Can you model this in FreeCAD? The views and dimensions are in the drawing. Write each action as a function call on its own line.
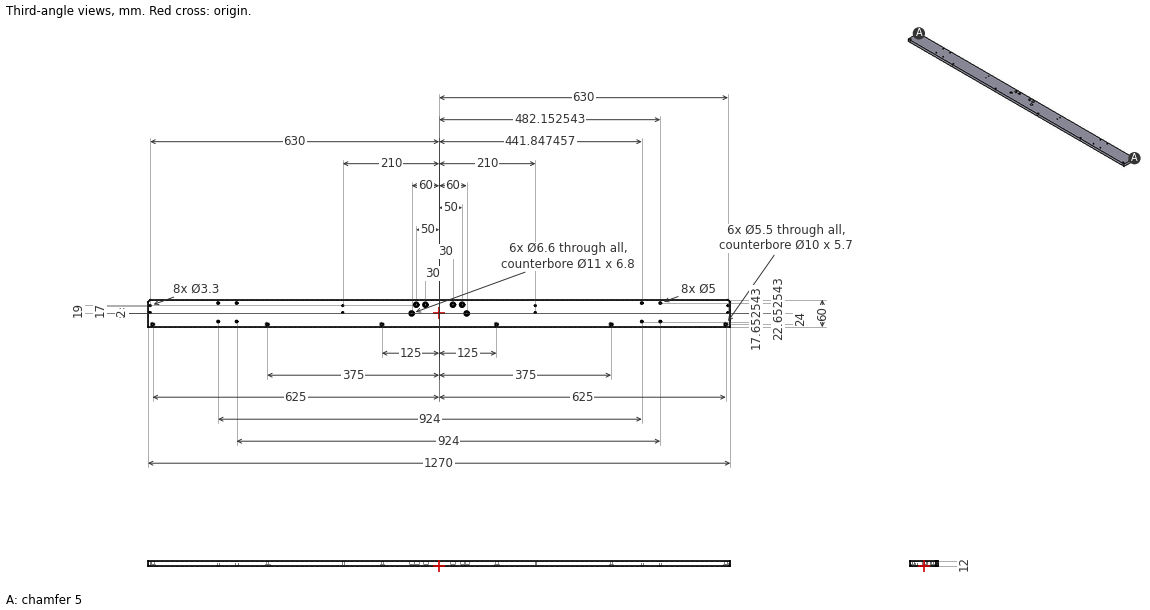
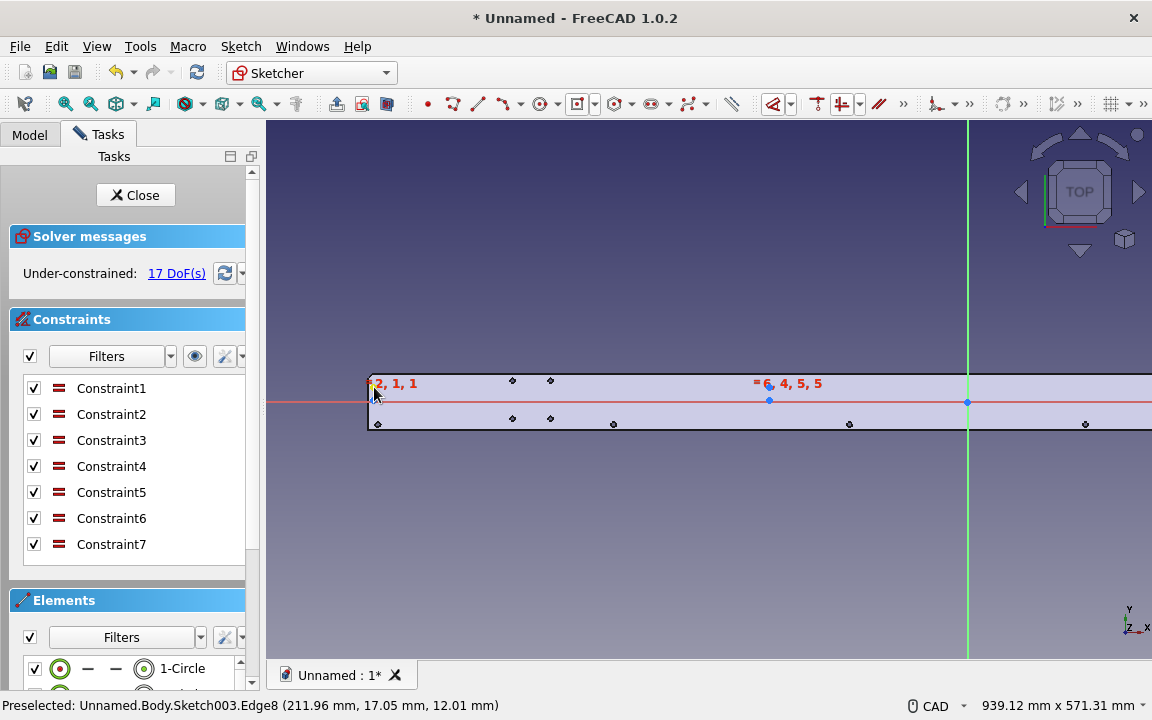
click(373, 387)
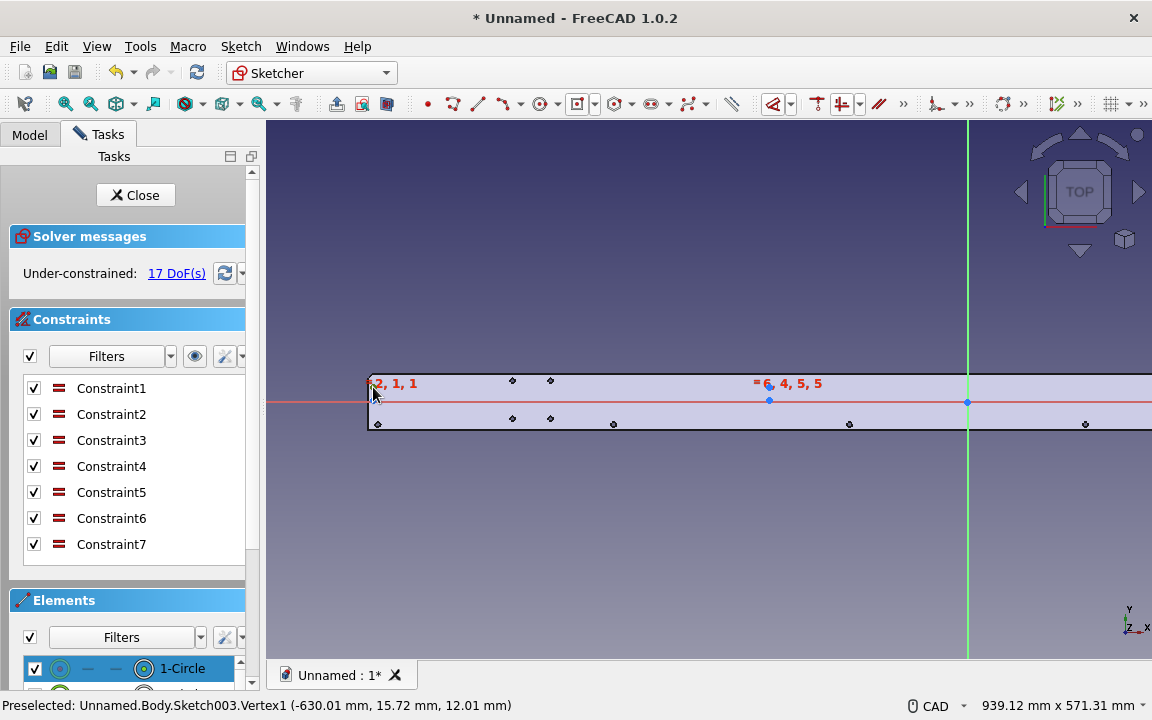
click(373, 400)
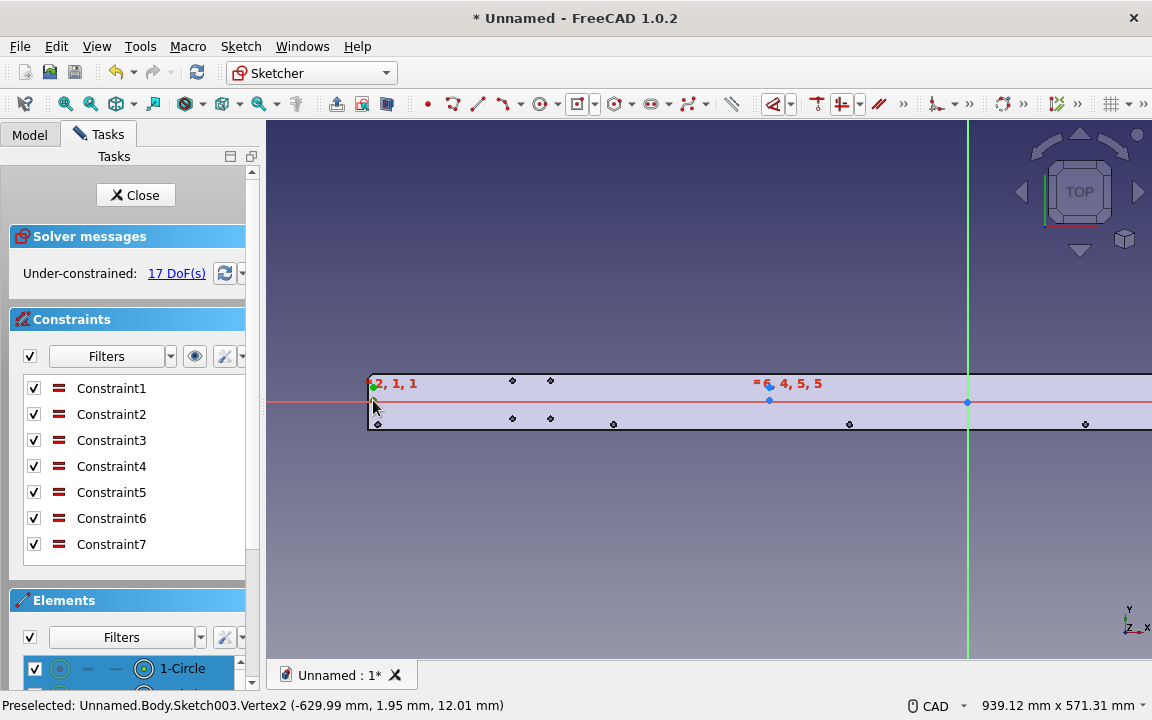
key(v)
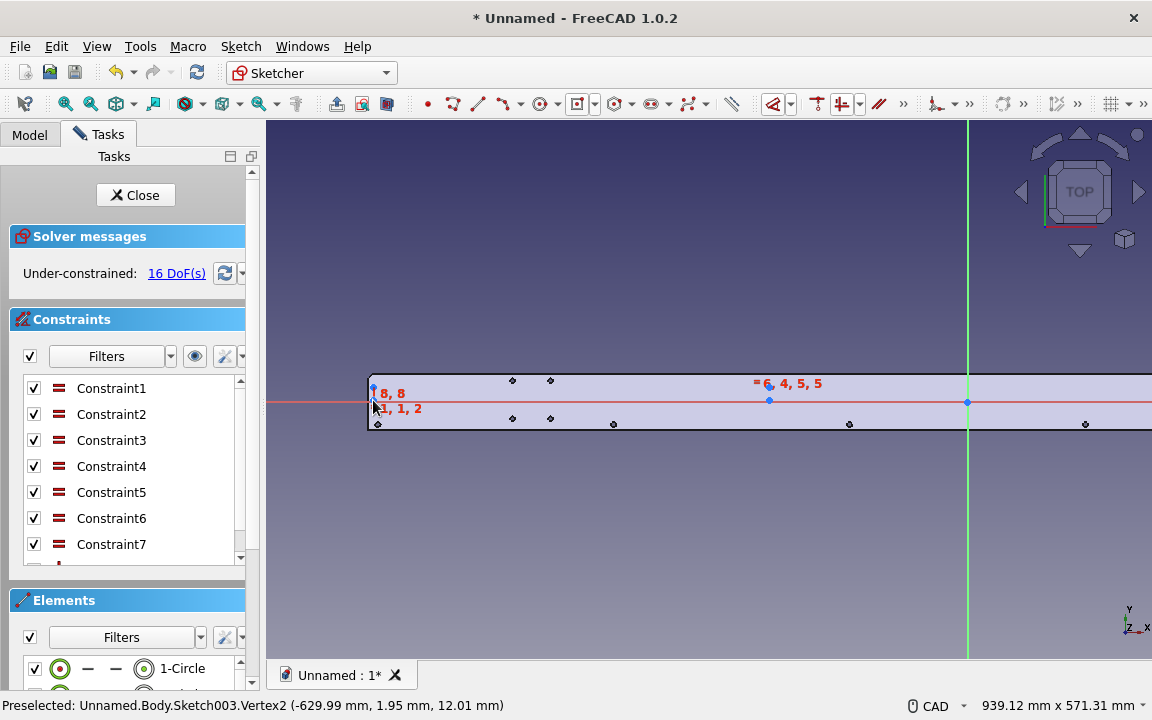
scroll(373, 400, up, 4)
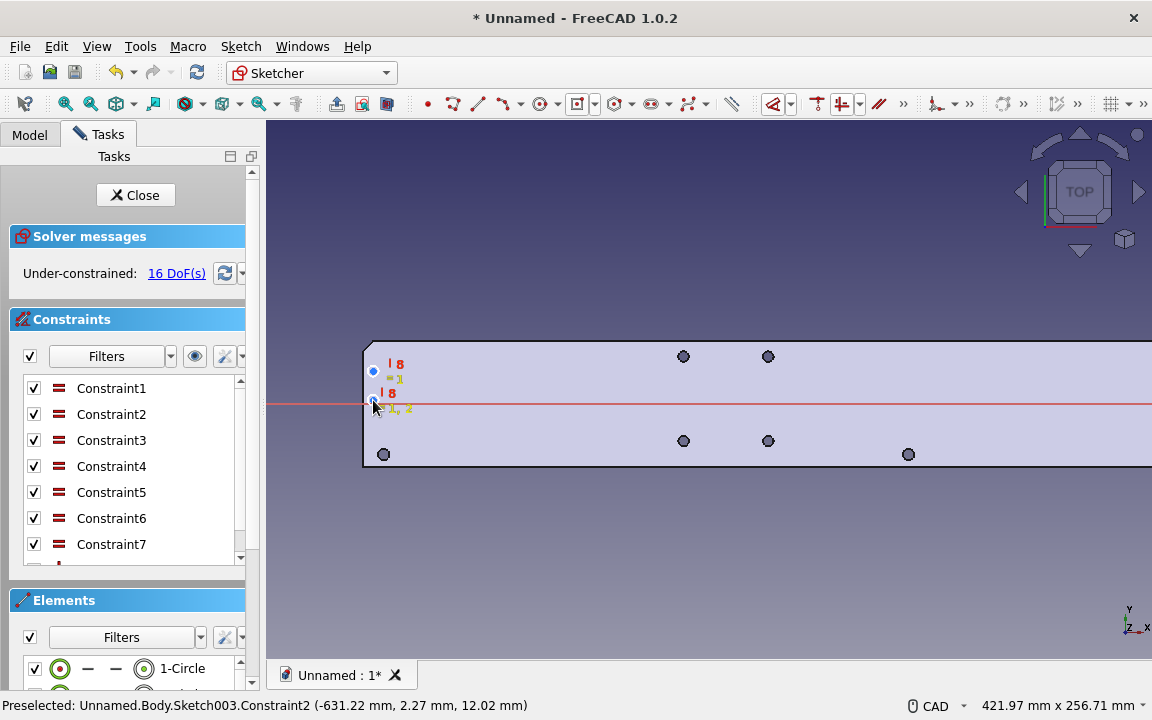
click(373, 400)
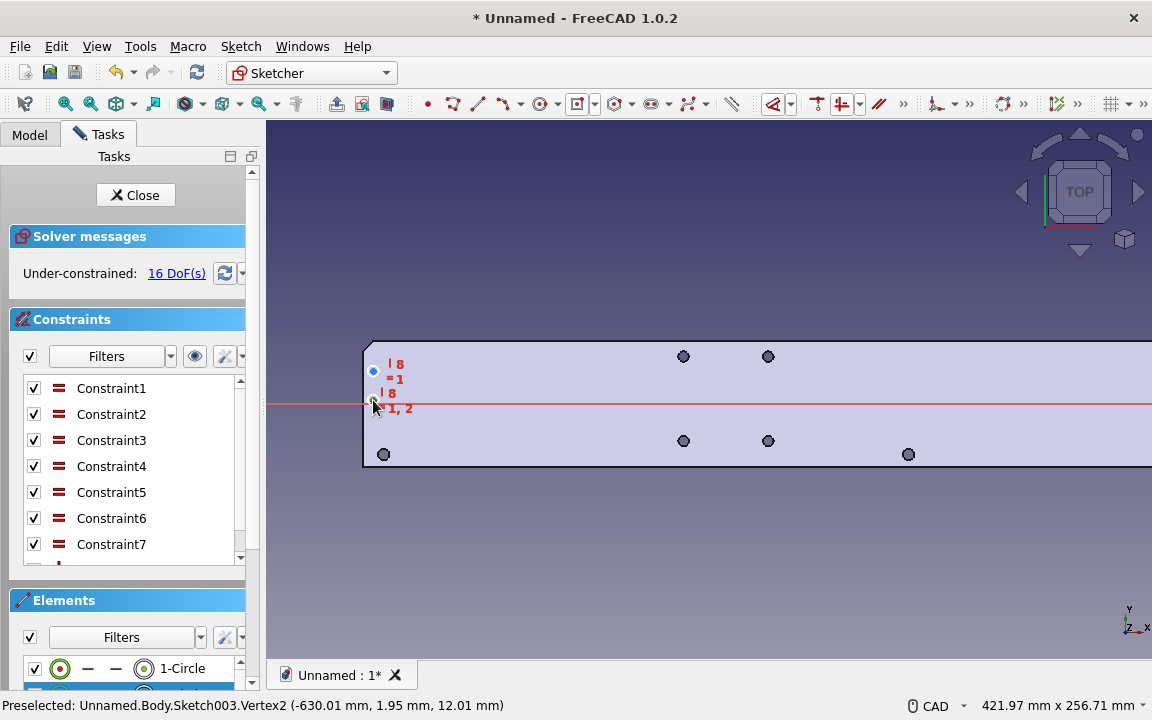
scroll(373, 391, down, 8)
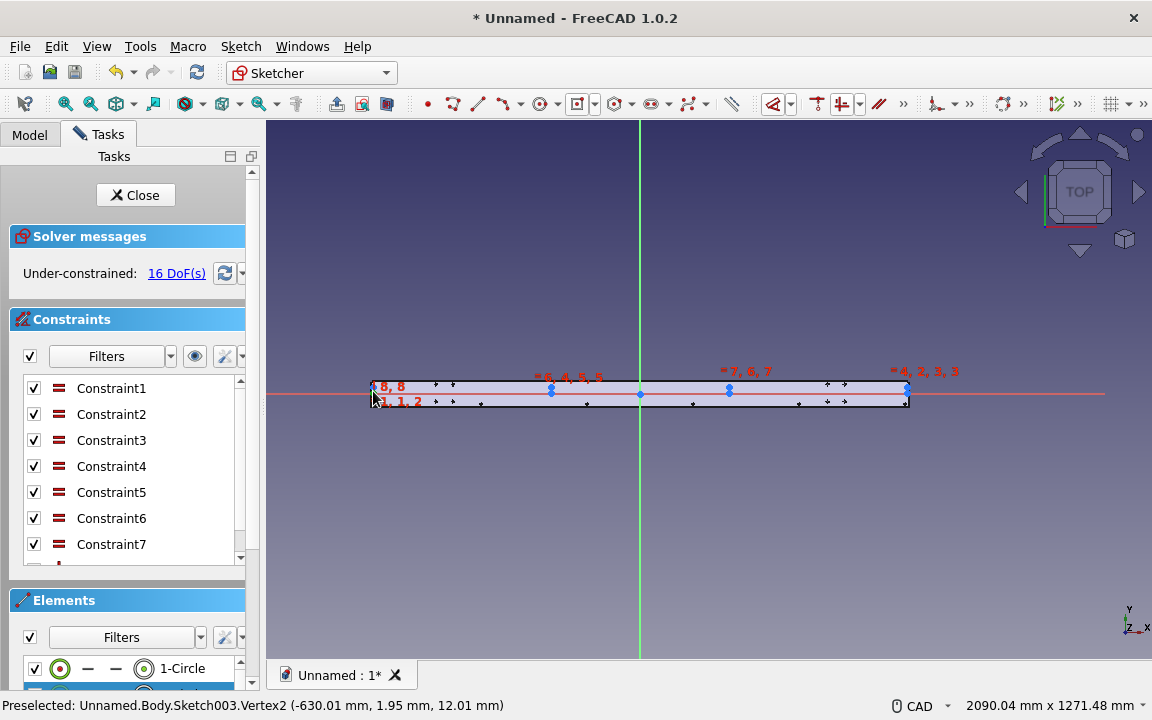
scroll(907, 393, up, 4)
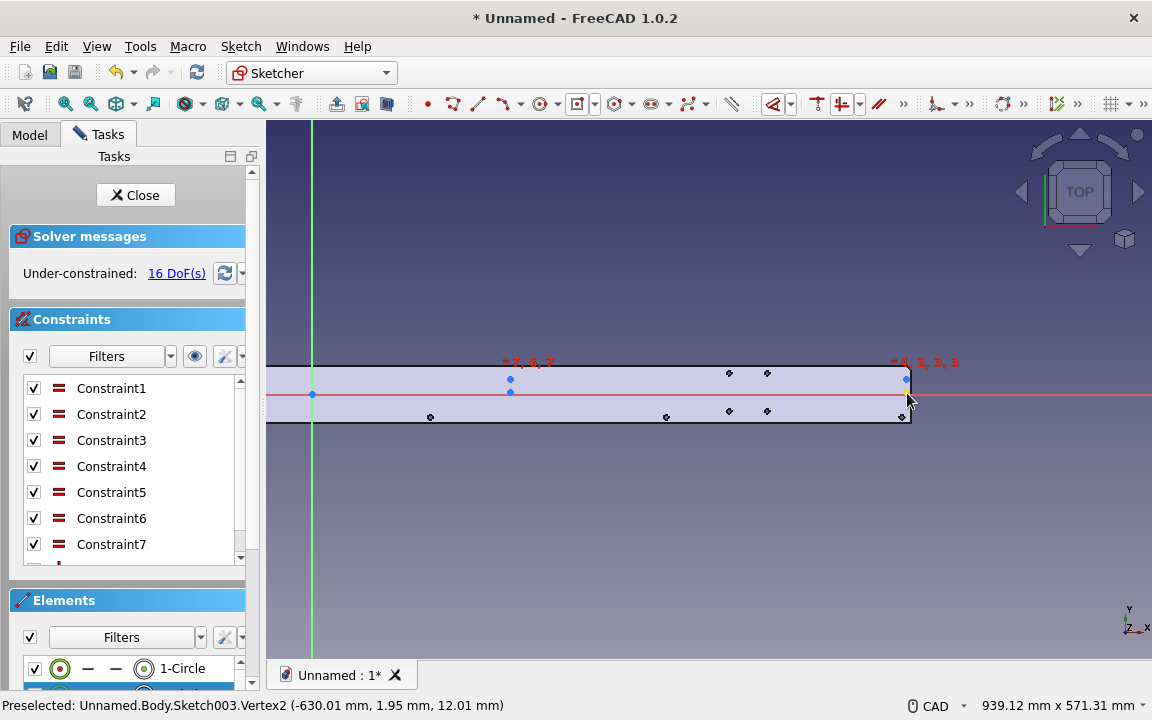
click(907, 393)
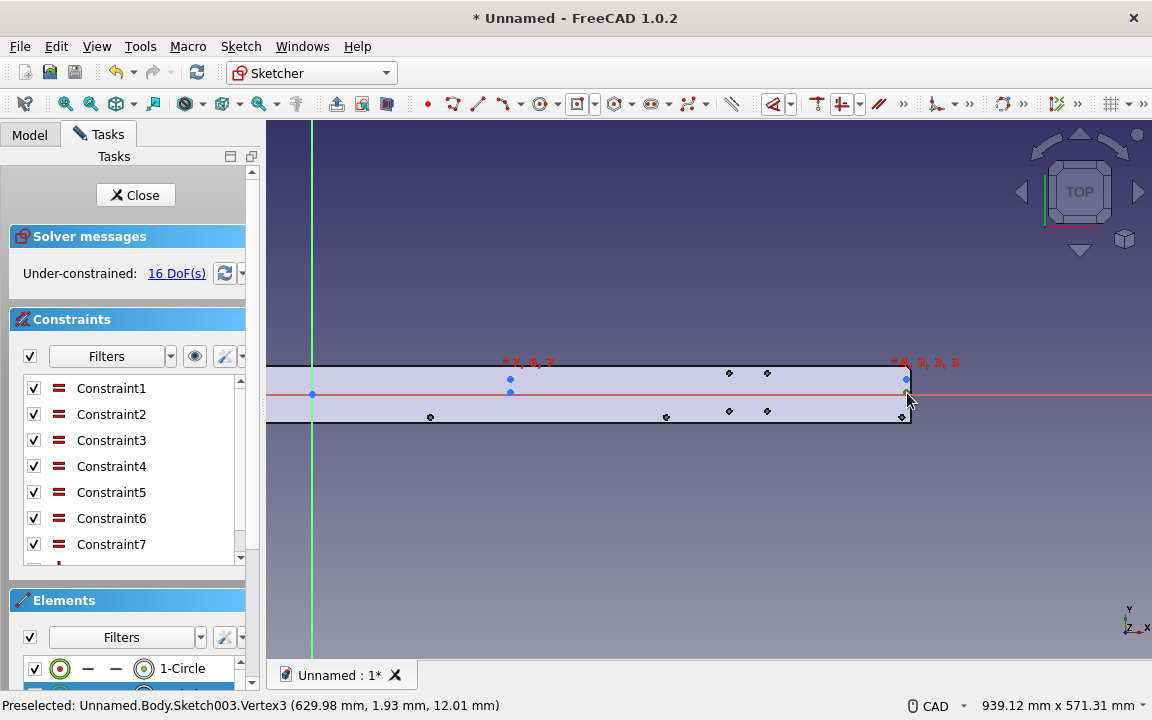
click(860, 104)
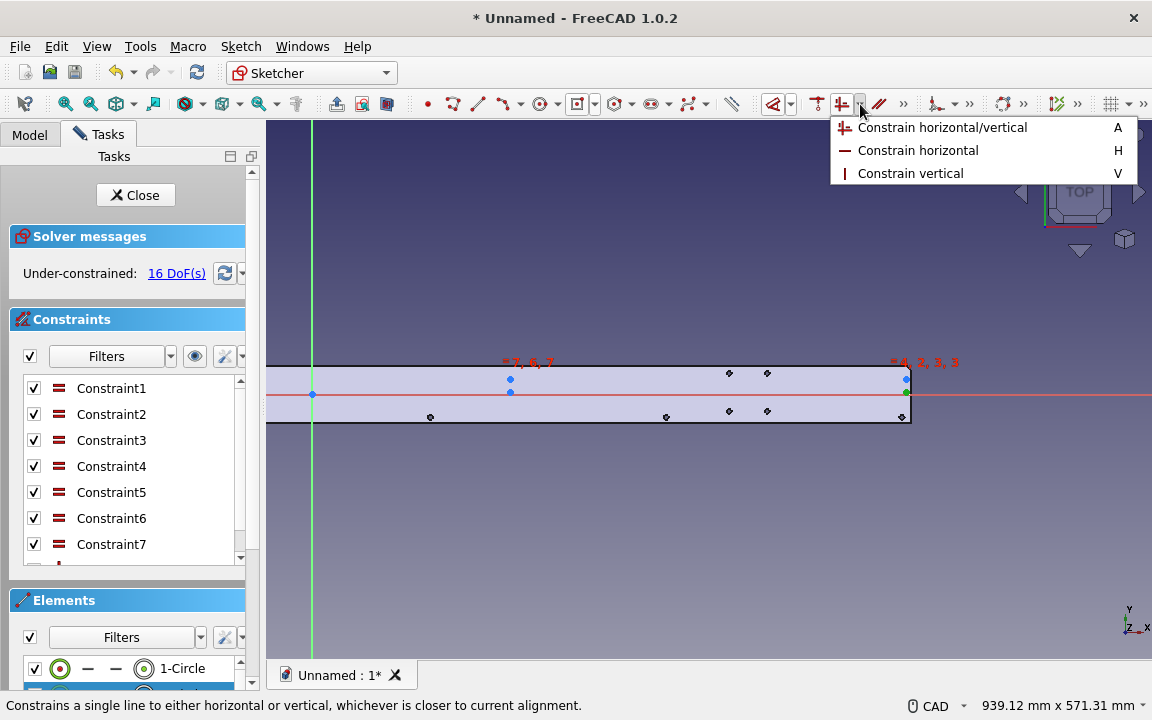
click(984, 150)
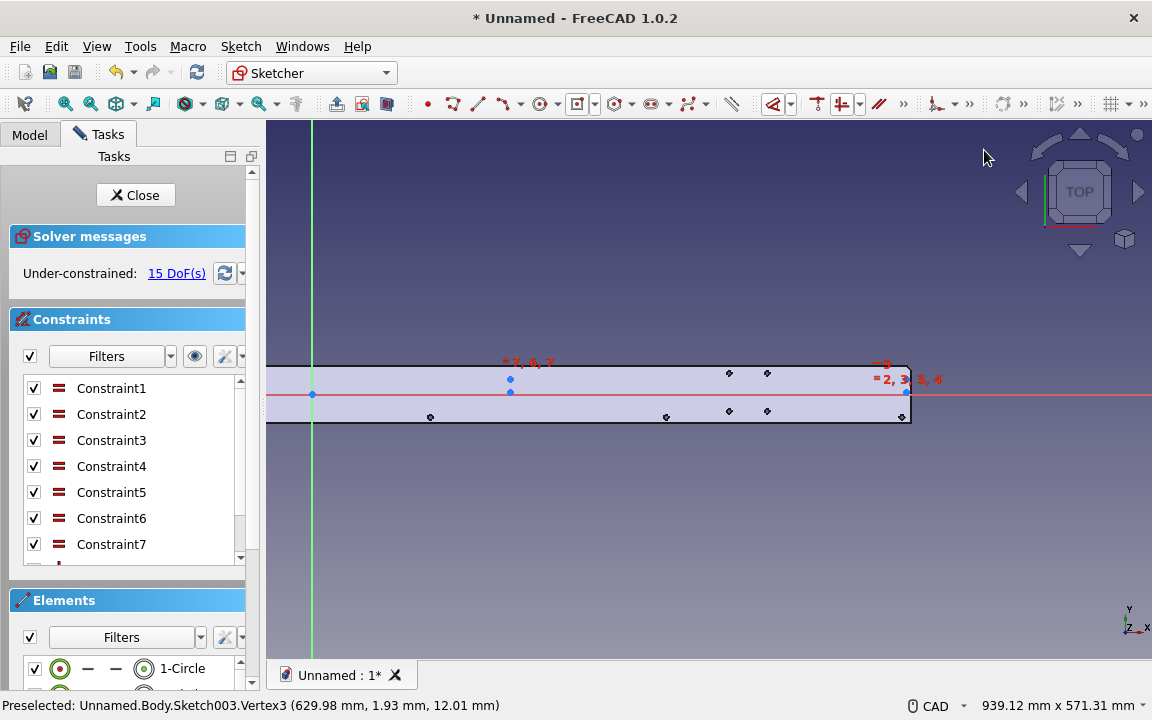
click(907, 393)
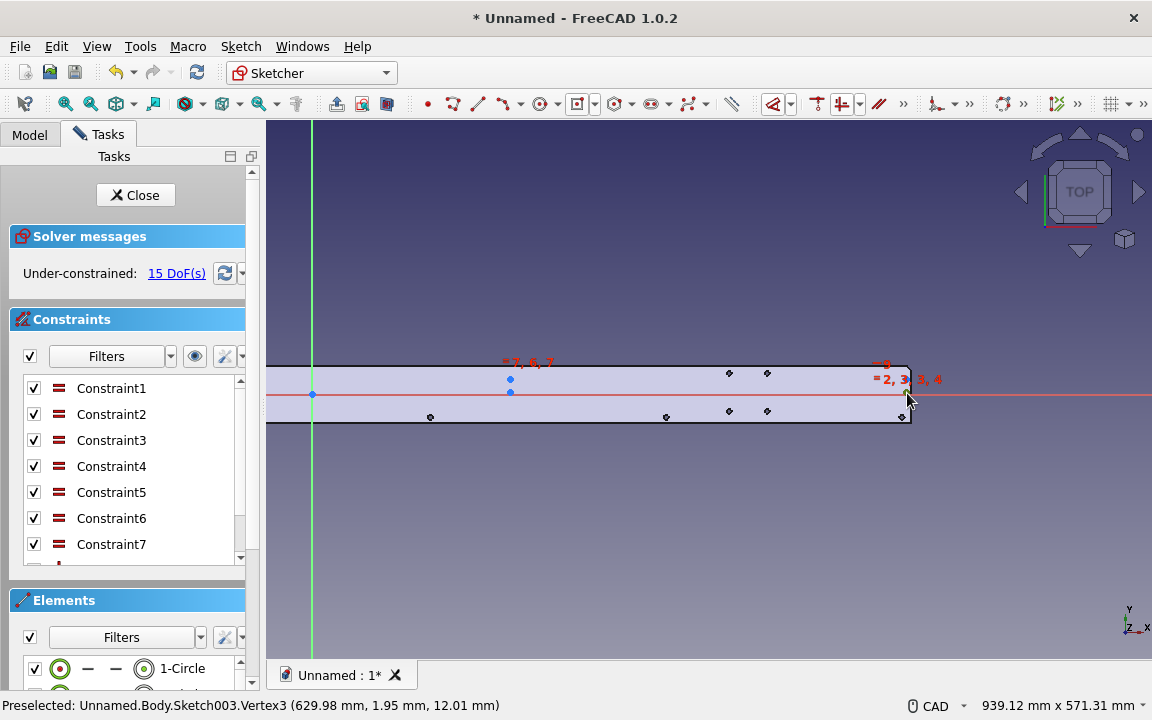
scroll(907, 379, up, 4)